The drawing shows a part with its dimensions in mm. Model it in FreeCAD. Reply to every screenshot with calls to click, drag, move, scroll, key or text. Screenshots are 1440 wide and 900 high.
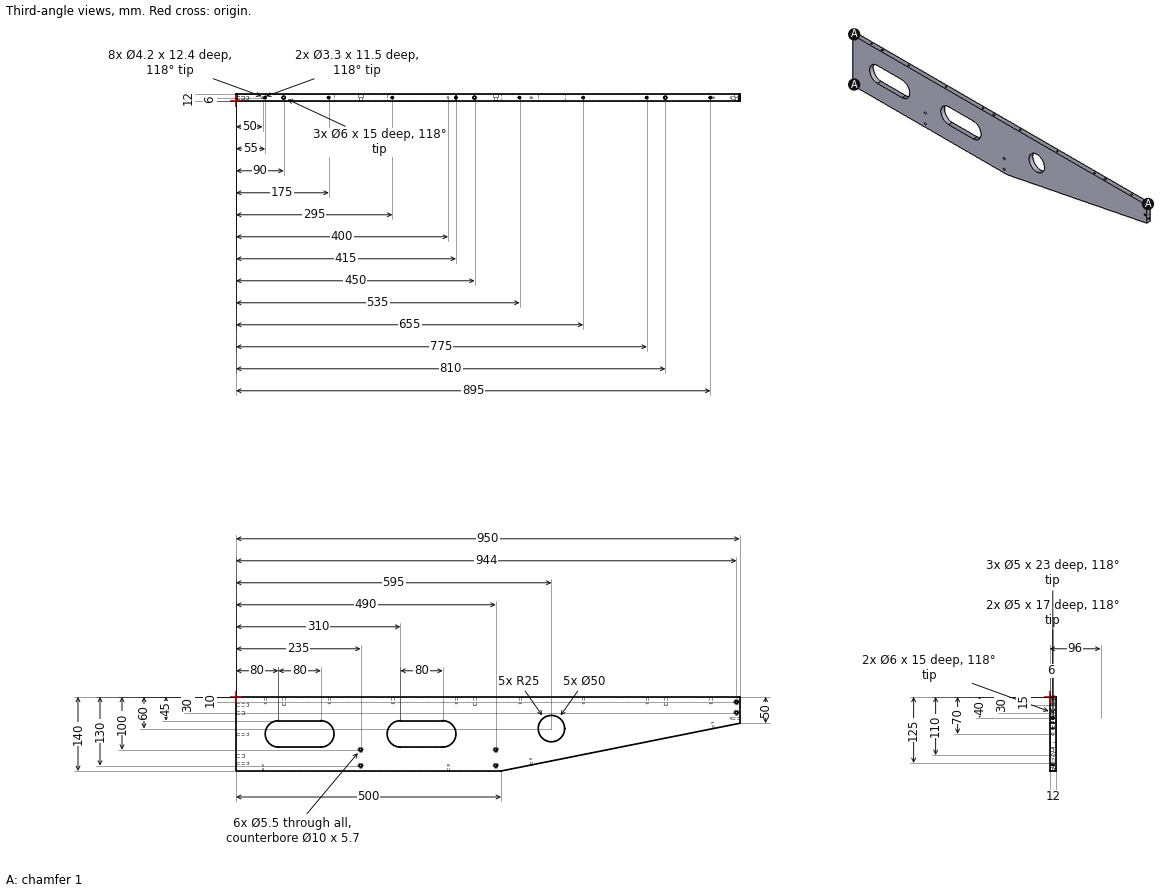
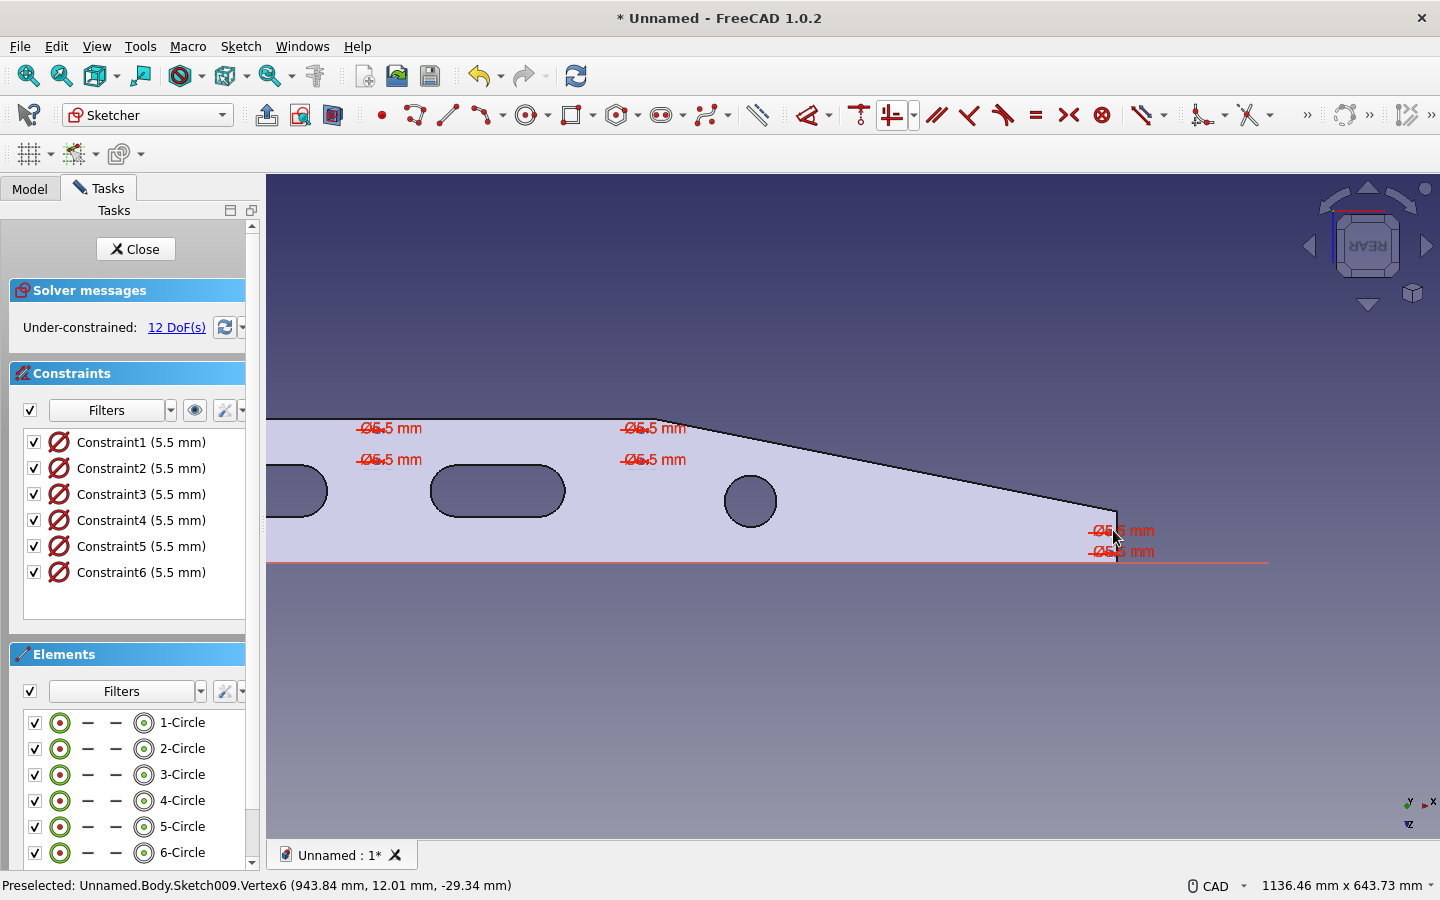
click(806, 116)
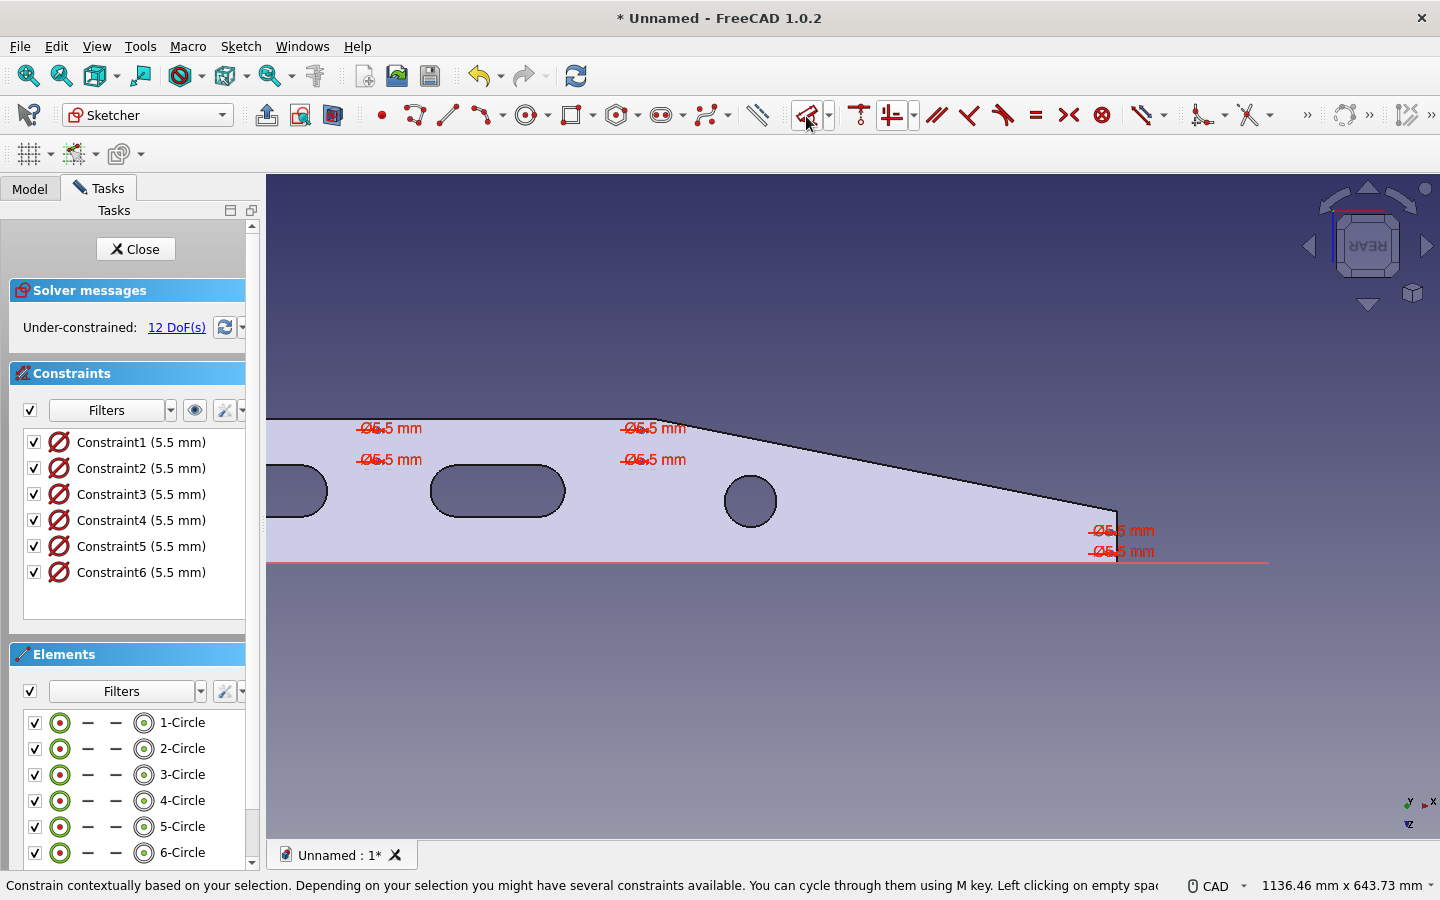
scroll(1111, 554, up, 7)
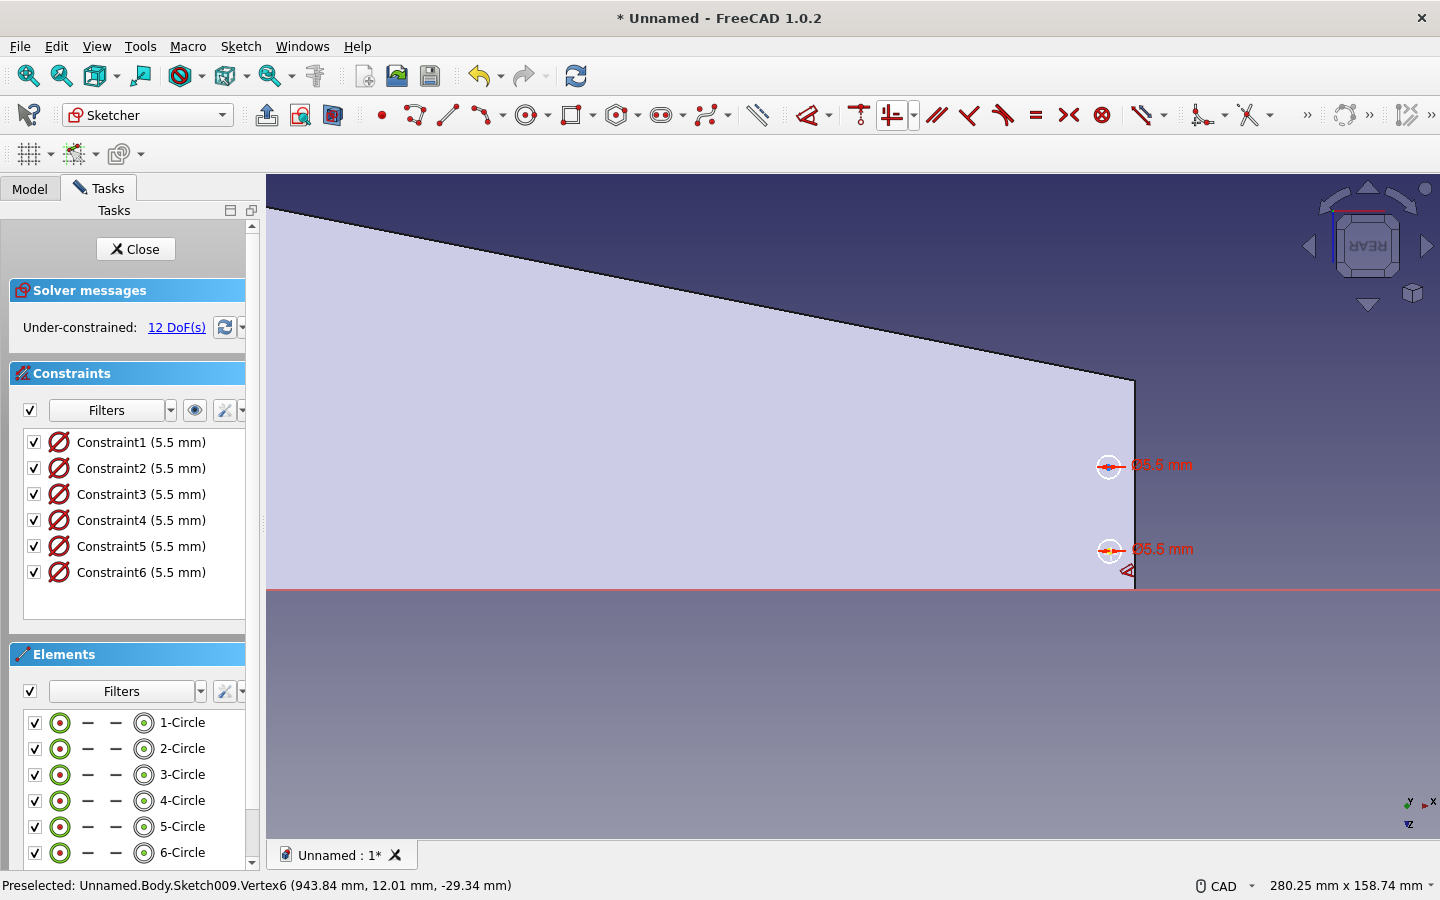
click(1110, 551)
click(1144, 571)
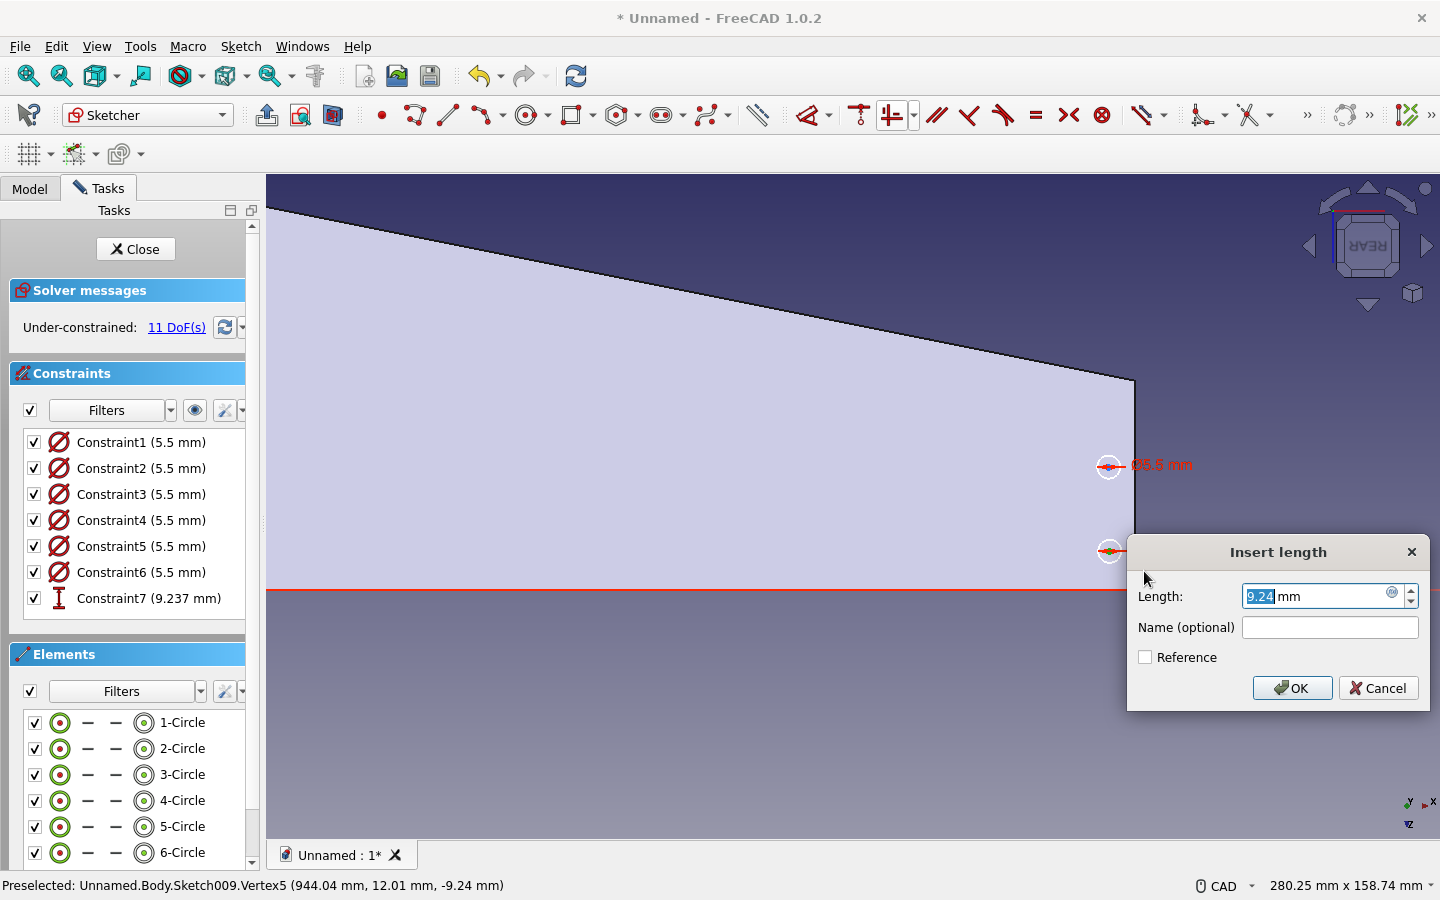
text(10)
key(Return)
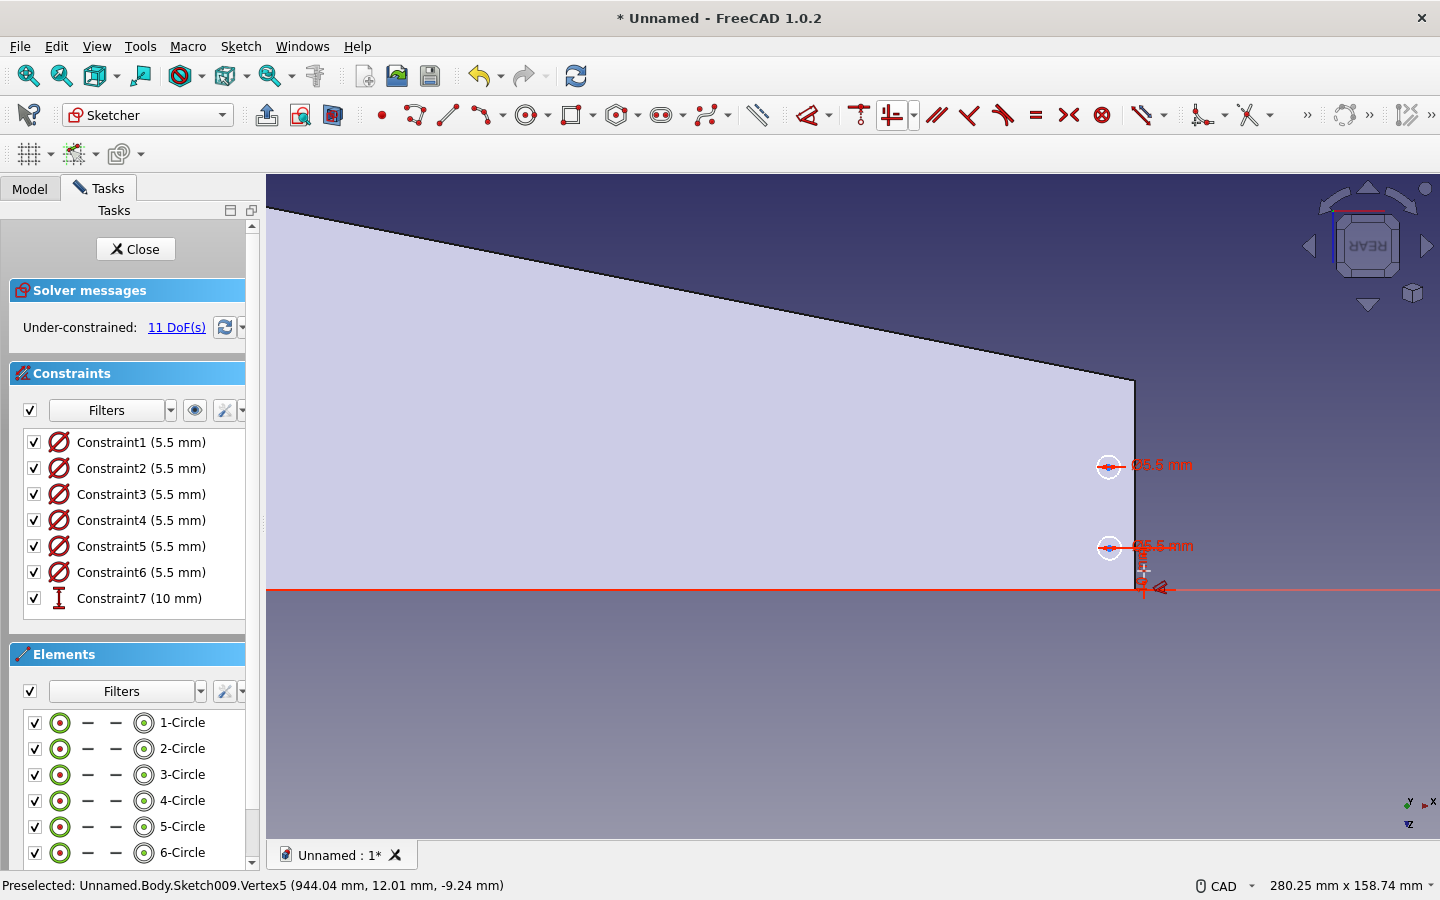
scroll(1111, 545, down, 9)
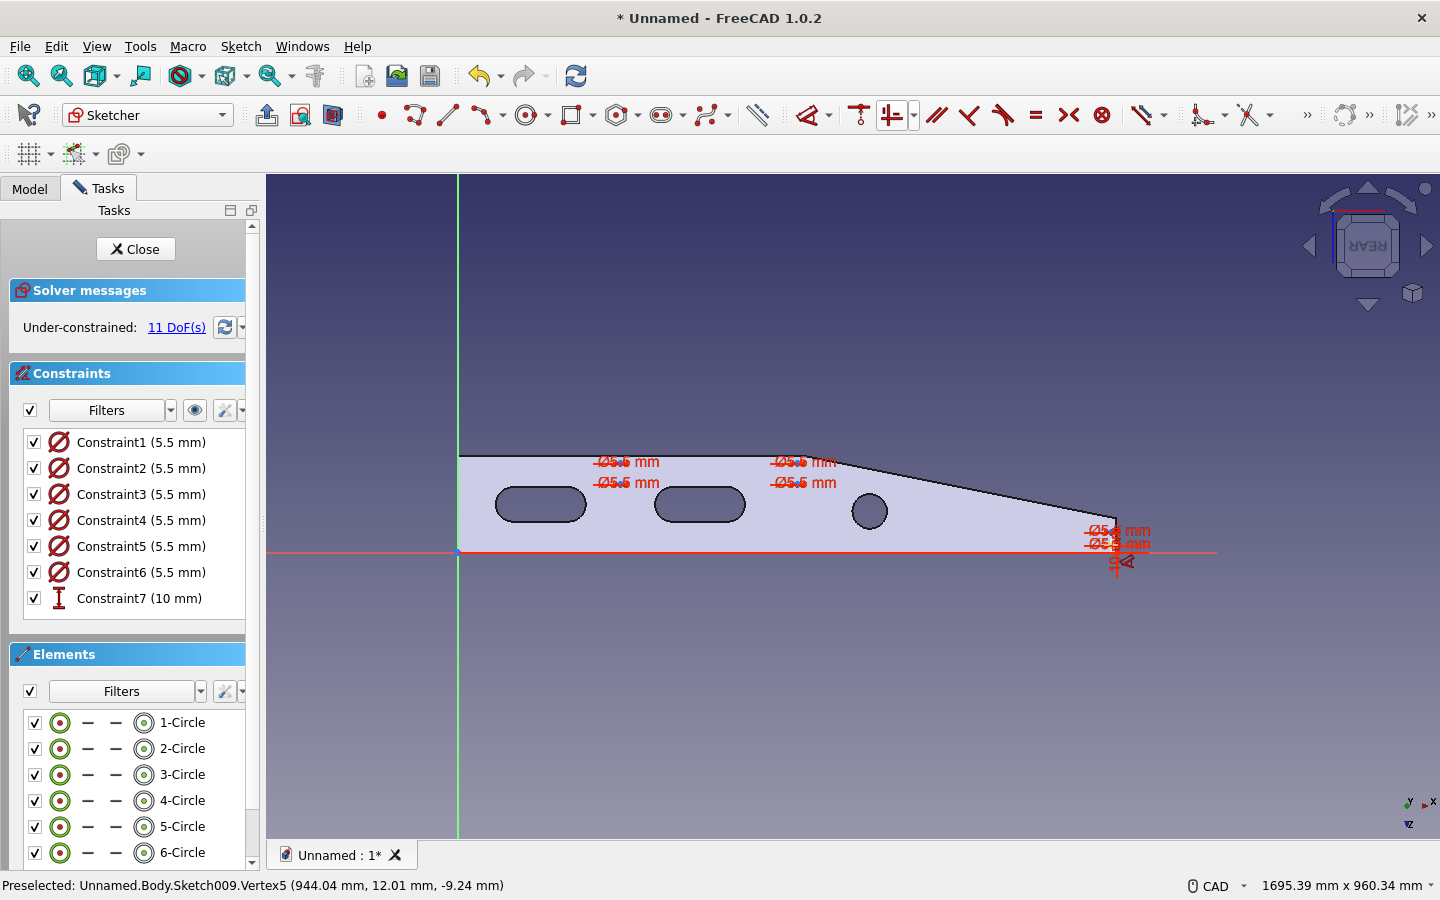
scroll(1111, 533, up, 4)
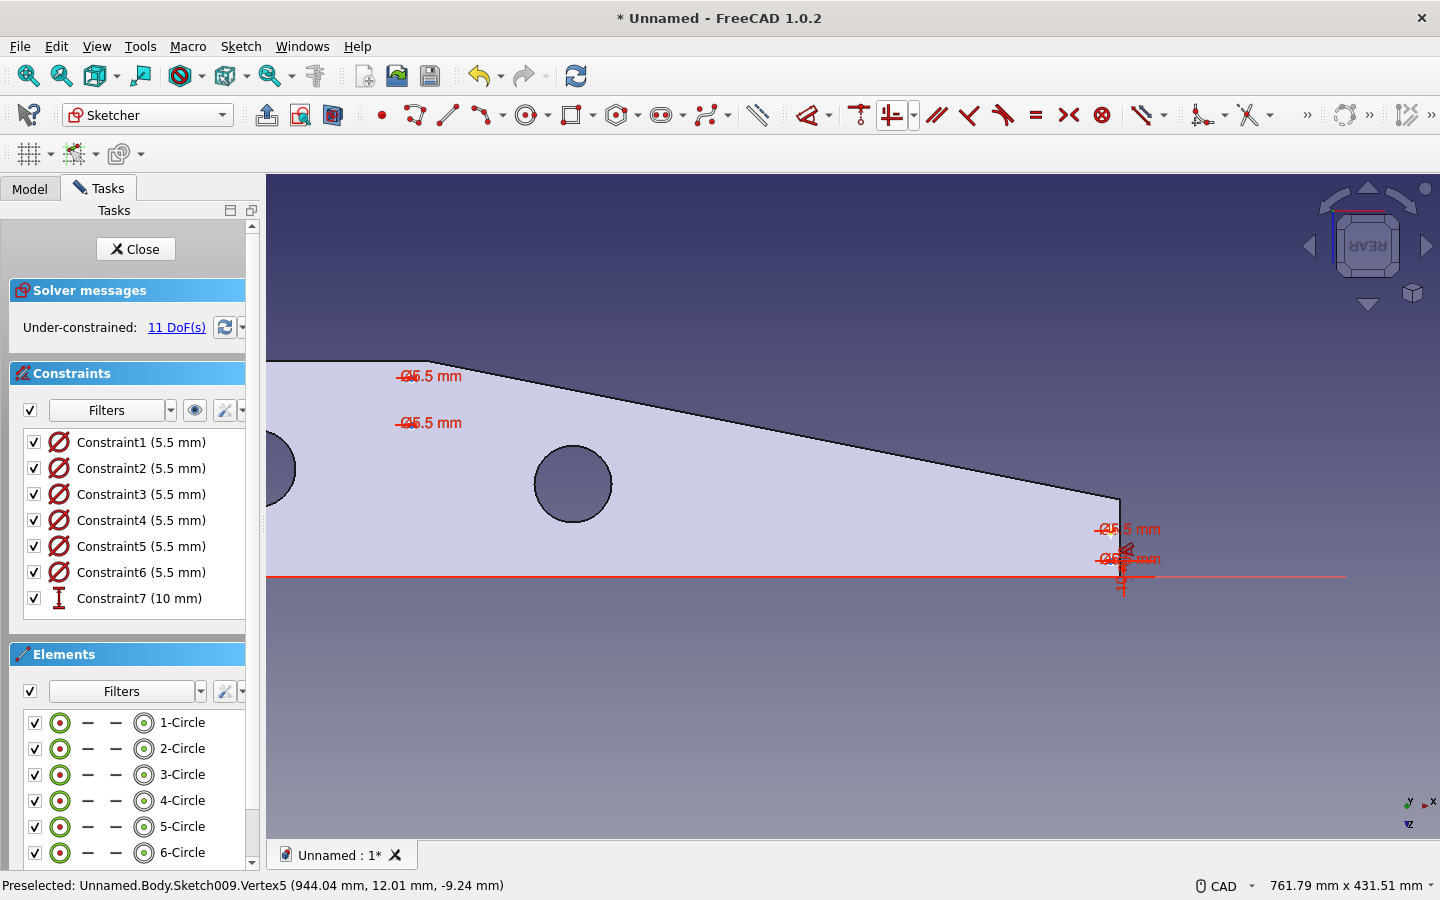
click(1111, 531)
click(1145, 544)